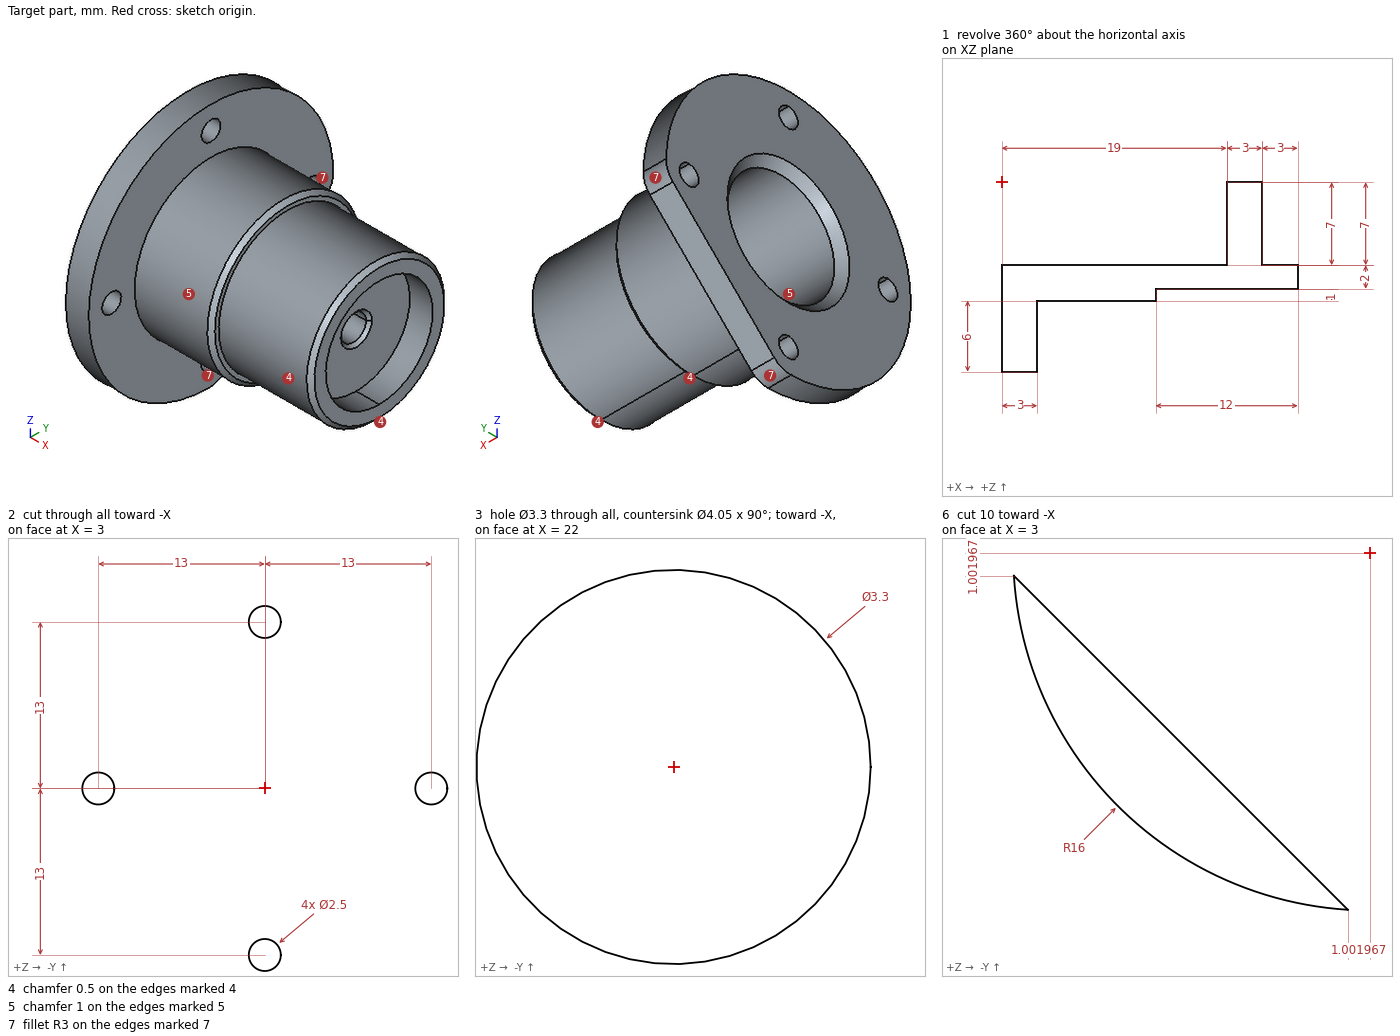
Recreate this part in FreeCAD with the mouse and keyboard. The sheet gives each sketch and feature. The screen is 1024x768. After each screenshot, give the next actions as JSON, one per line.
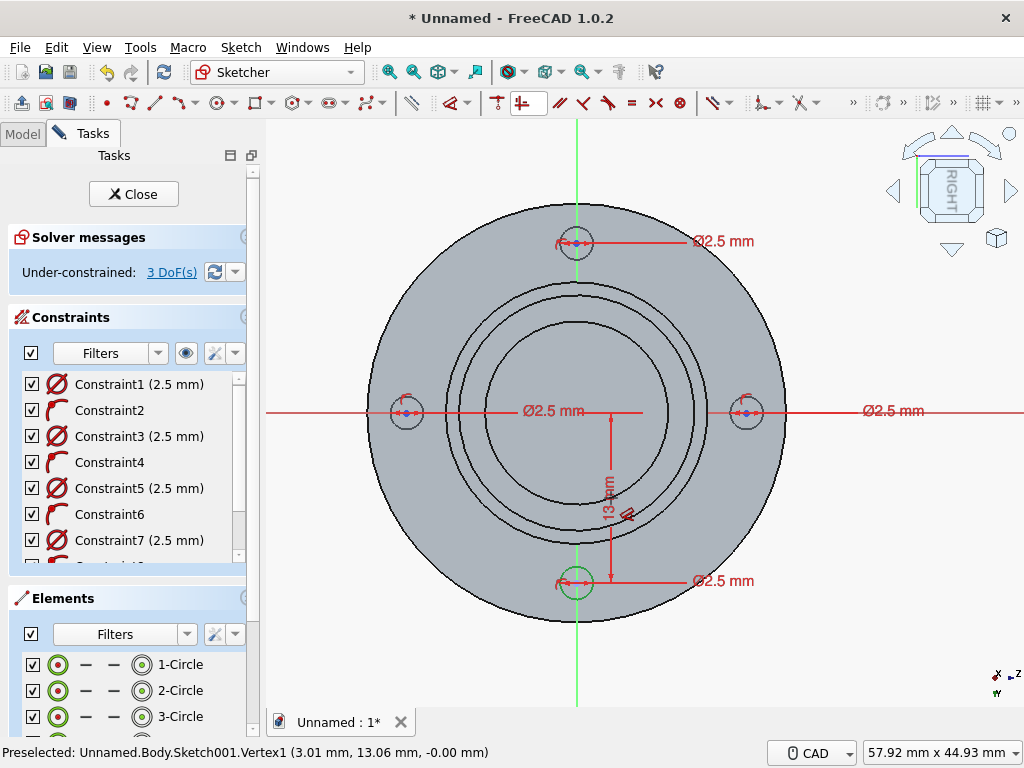
{"action": "left_click", "coordinate": [407, 413]}
{"action": "left_click", "coordinate": [492, 447]}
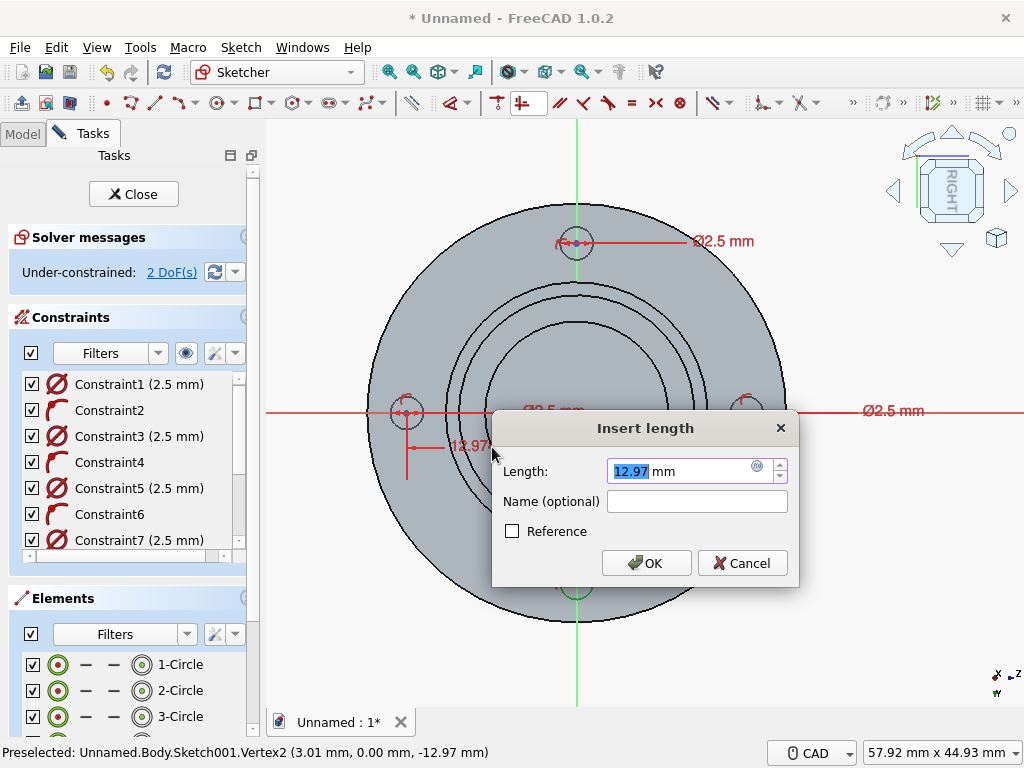
{"action": "type", "text": "13"}
{"action": "key", "text": "Return"}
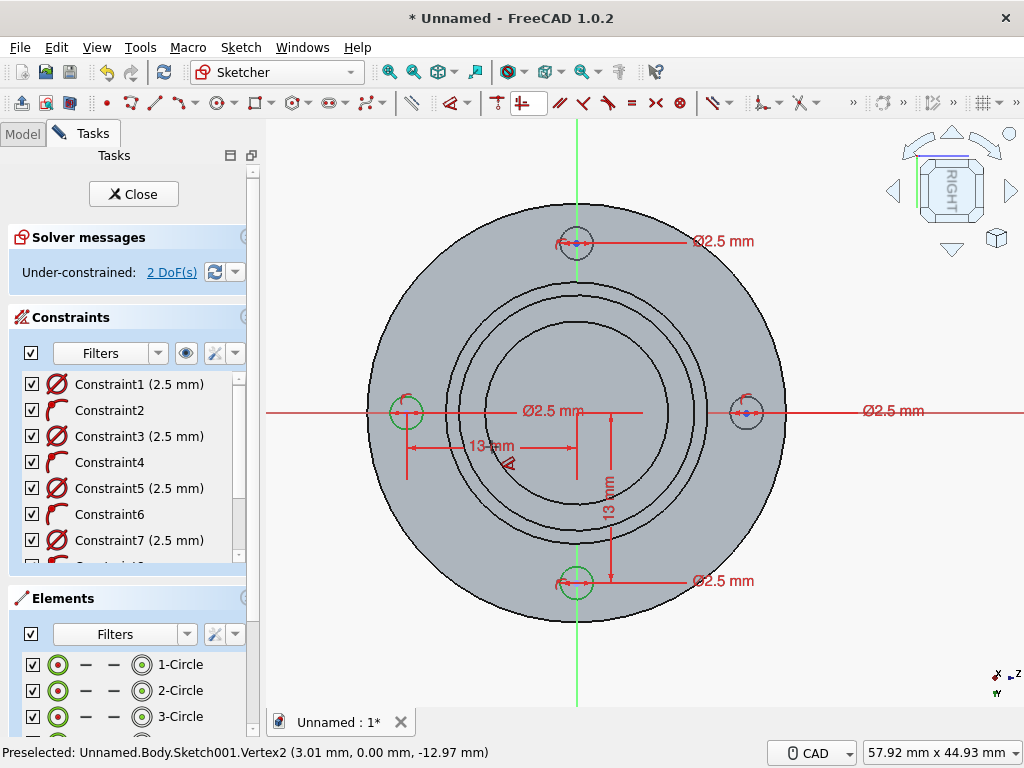
{"action": "left_click", "coordinate": [577, 243]}
{"action": "left_click", "coordinate": [611, 328]}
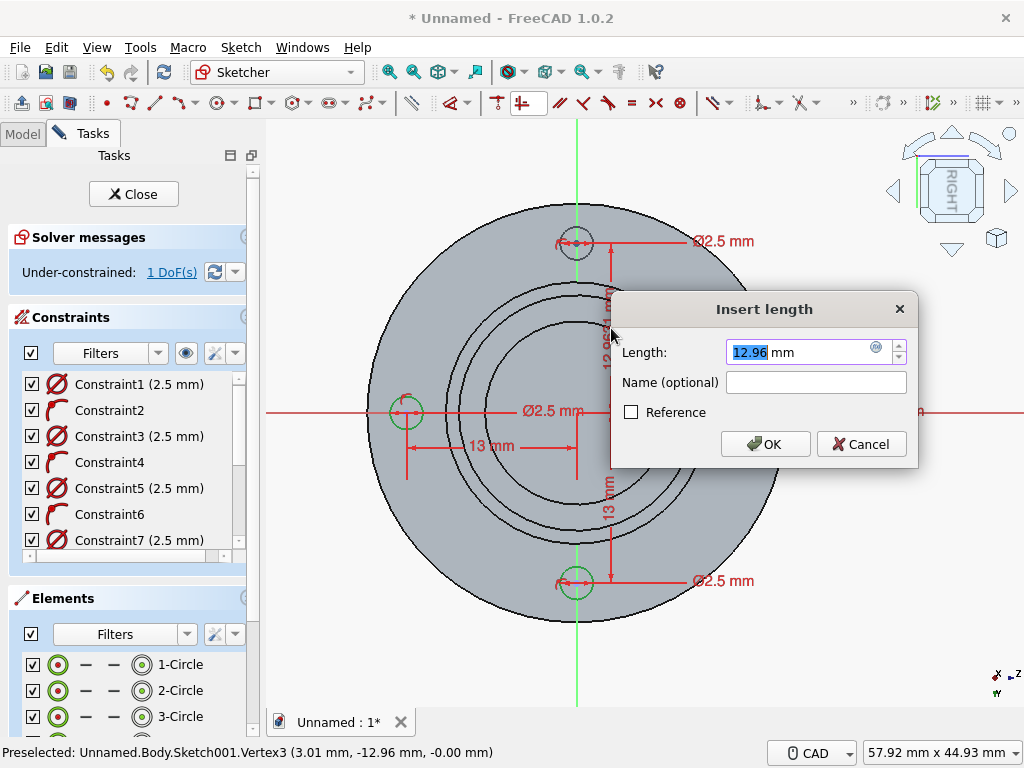
{"action": "type", "text": "13"}
{"action": "key", "text": "Return"}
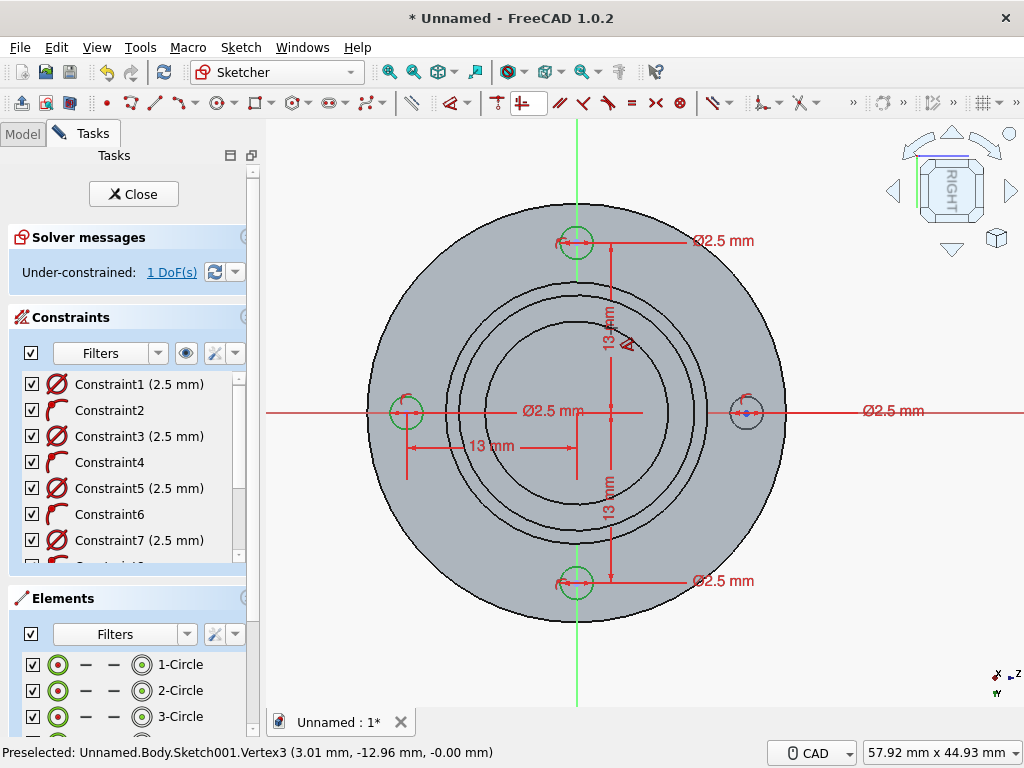
{"action": "left_click", "coordinate": [747, 413]}
{"action": "left_click", "coordinate": [662, 447]}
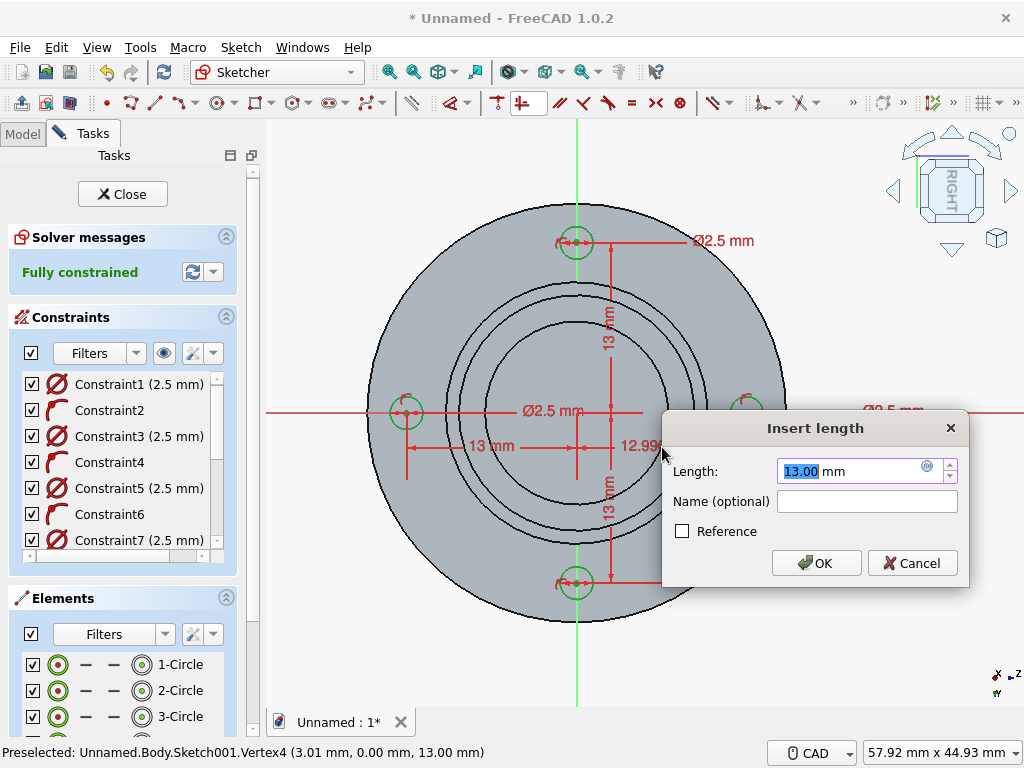
{"action": "type", "text": "13"}
{"action": "key", "text": "Return"}
{"action": "key", "text": "Escape"}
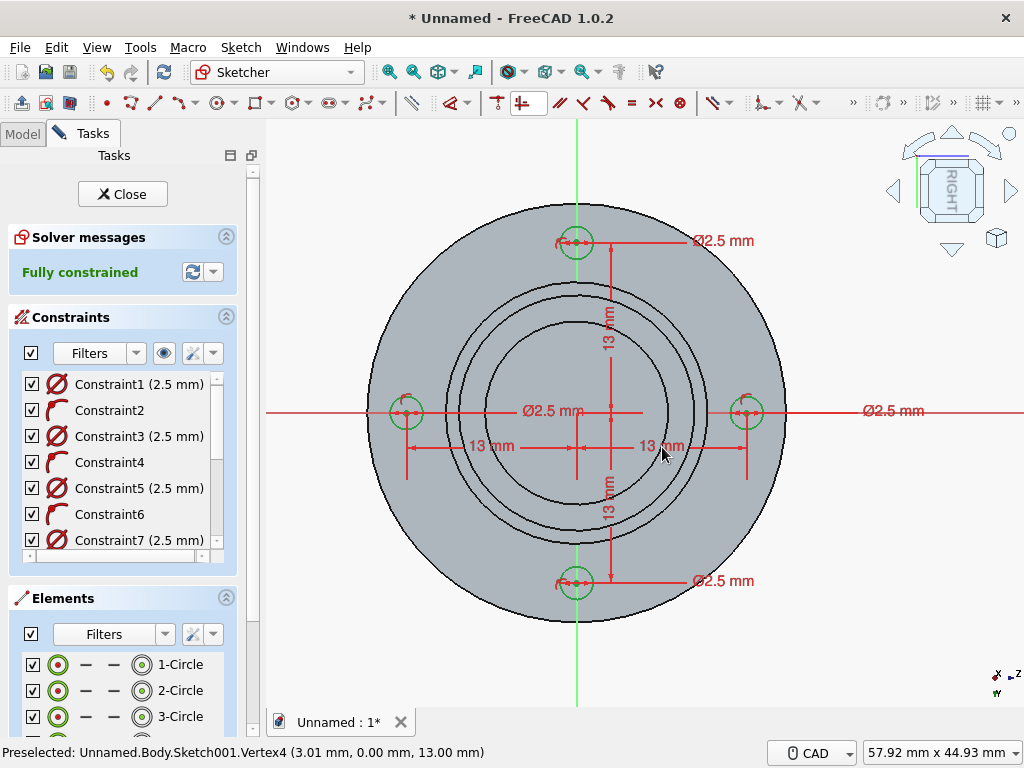
{"action": "left_click", "coordinate": [123, 194]}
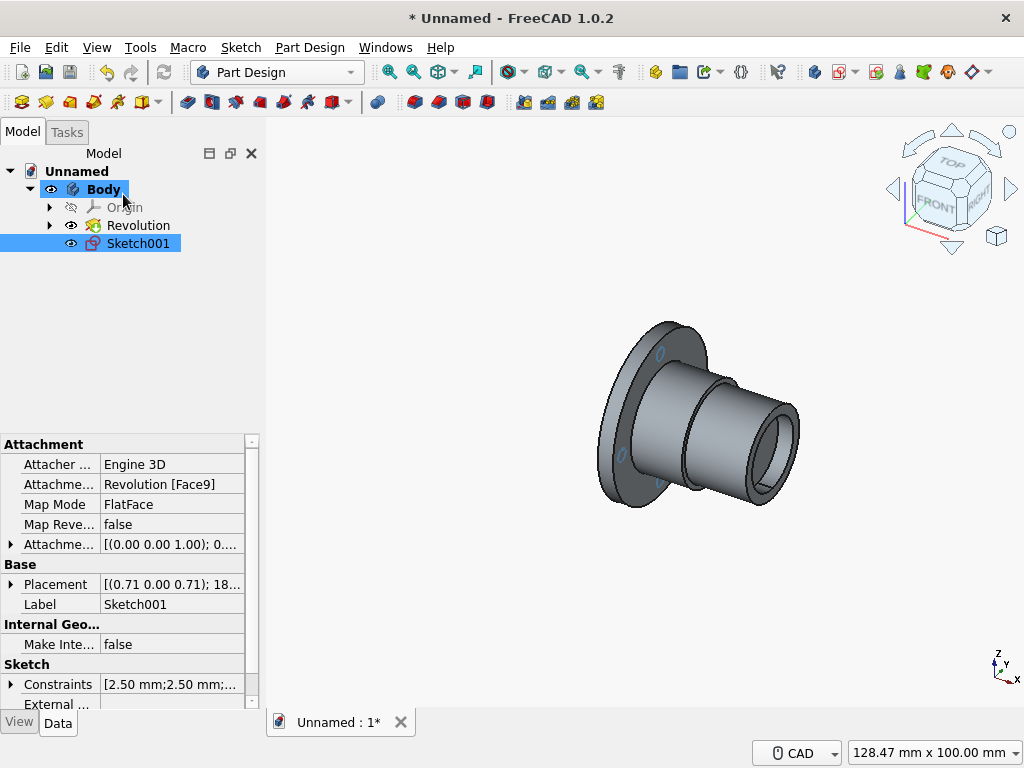
{"action": "left_click", "coordinate": [188, 102]}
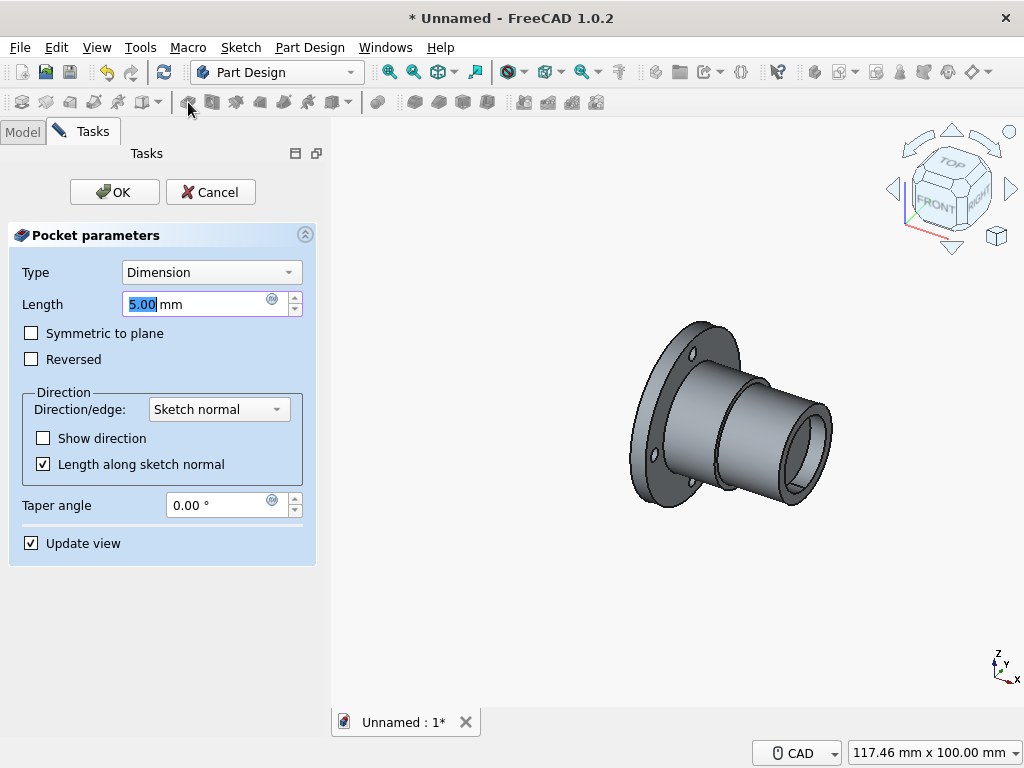
{"action": "left_click", "coordinate": [212, 272]}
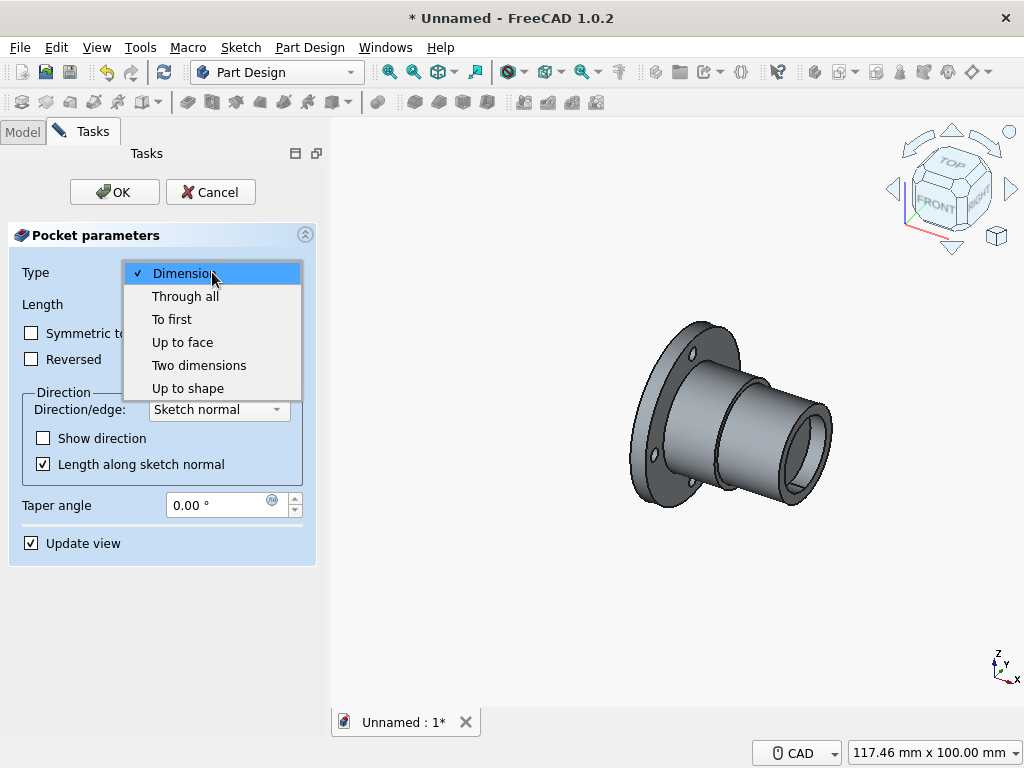
{"action": "left_click", "coordinate": [212, 296]}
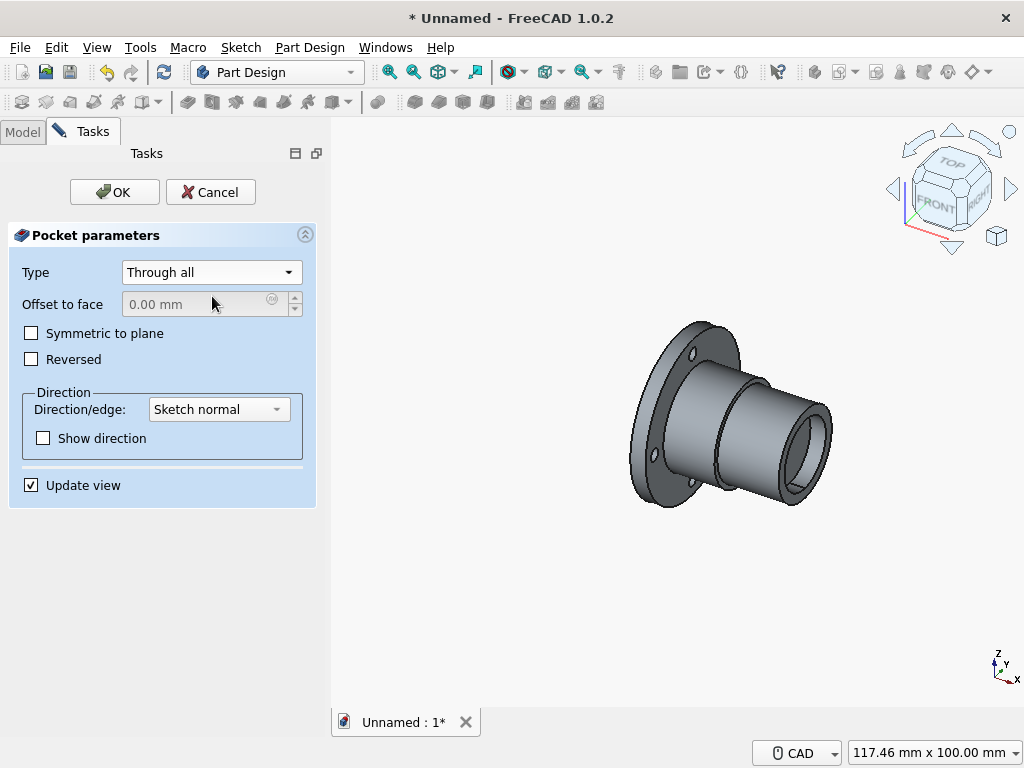
{"action": "left_click", "coordinate": [115, 192]}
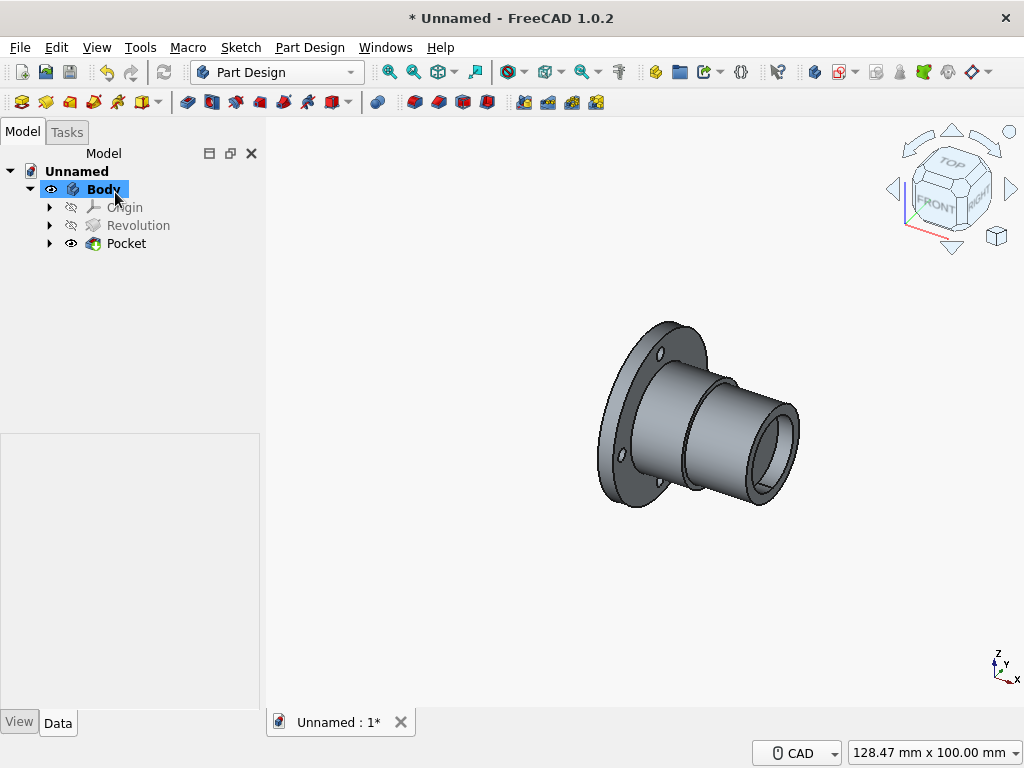
{"action": "key", "text": "0"}